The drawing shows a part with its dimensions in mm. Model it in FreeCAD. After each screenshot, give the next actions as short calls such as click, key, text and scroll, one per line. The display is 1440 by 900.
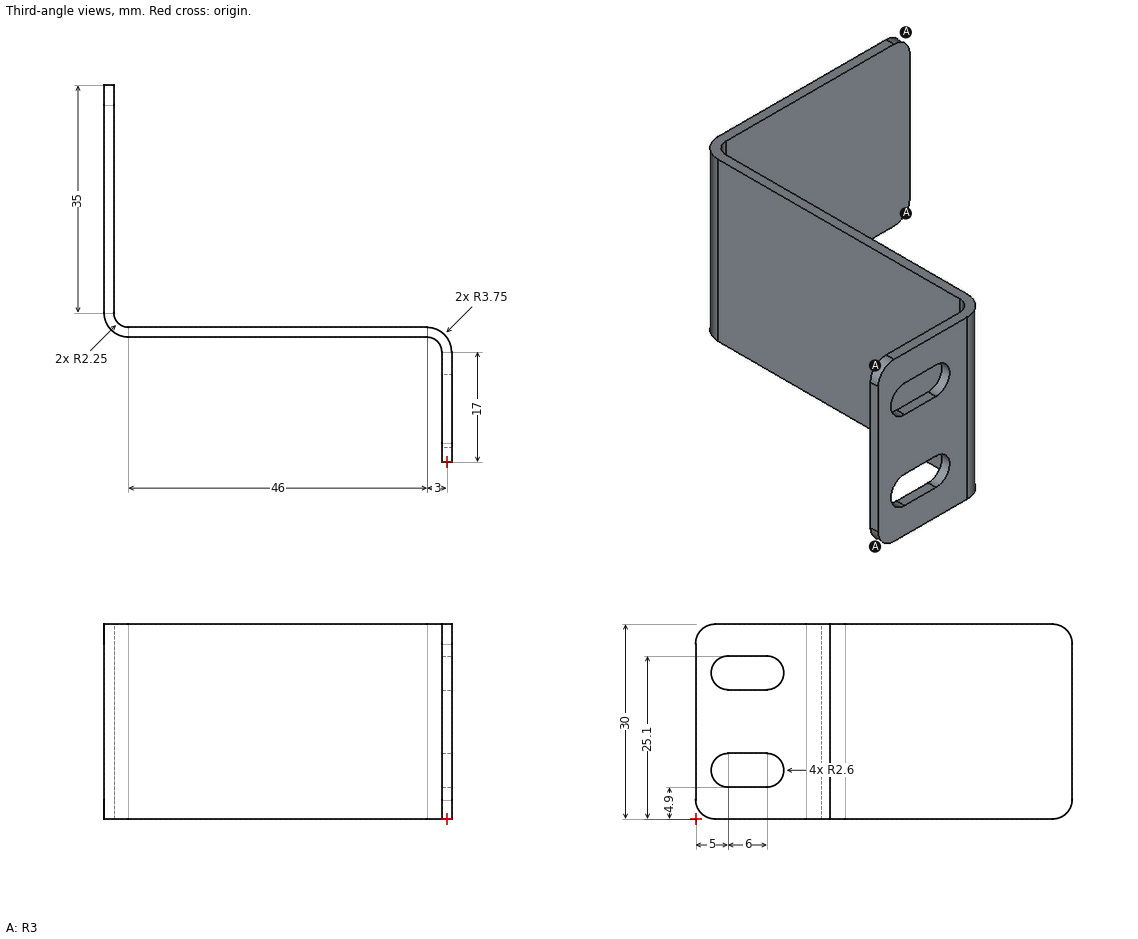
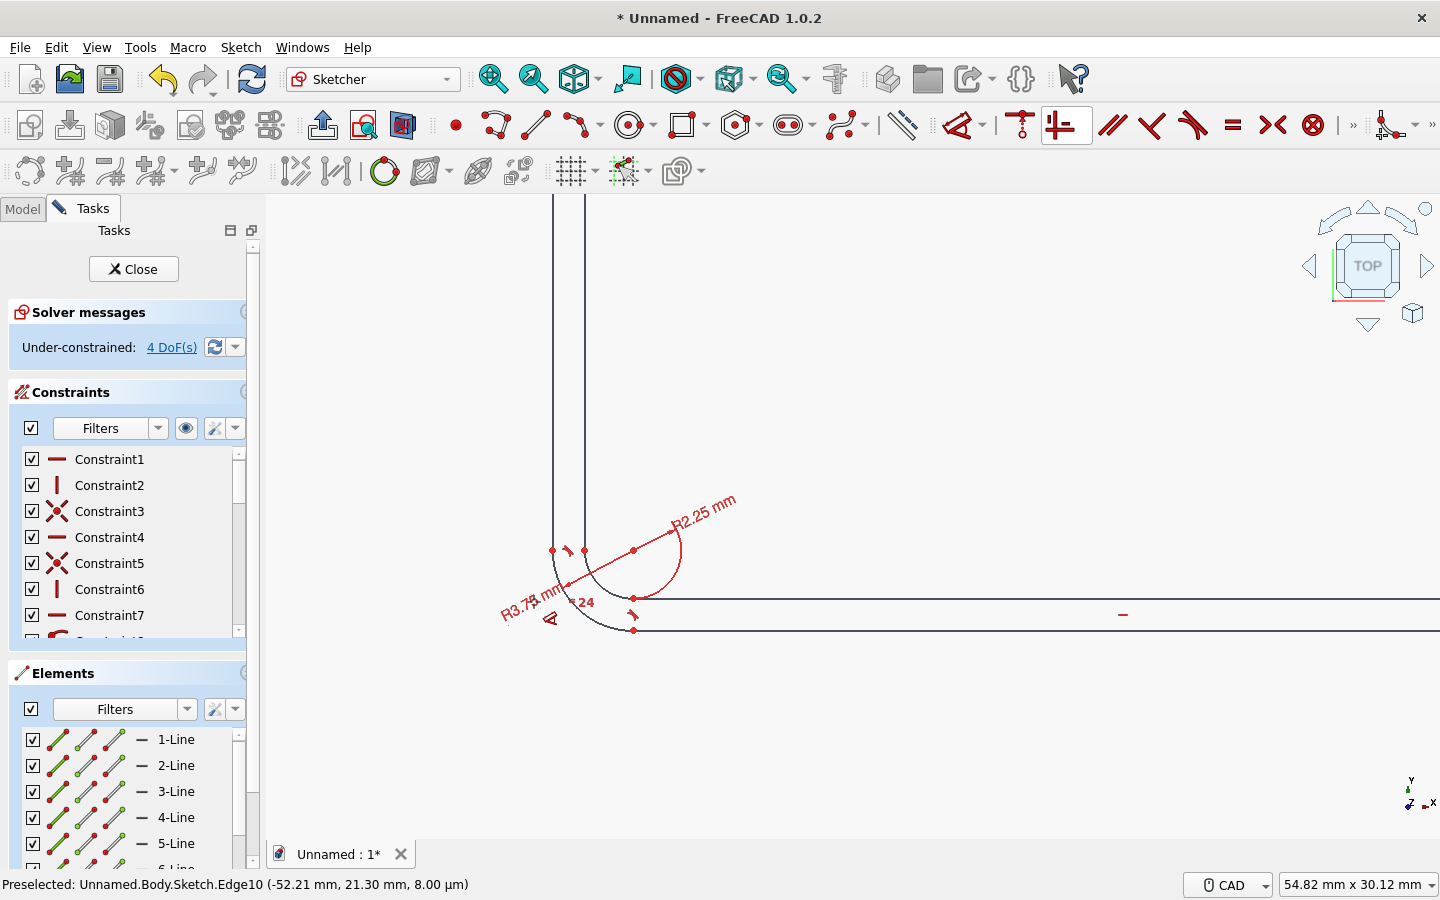
click(927, 599)
click(954, 565)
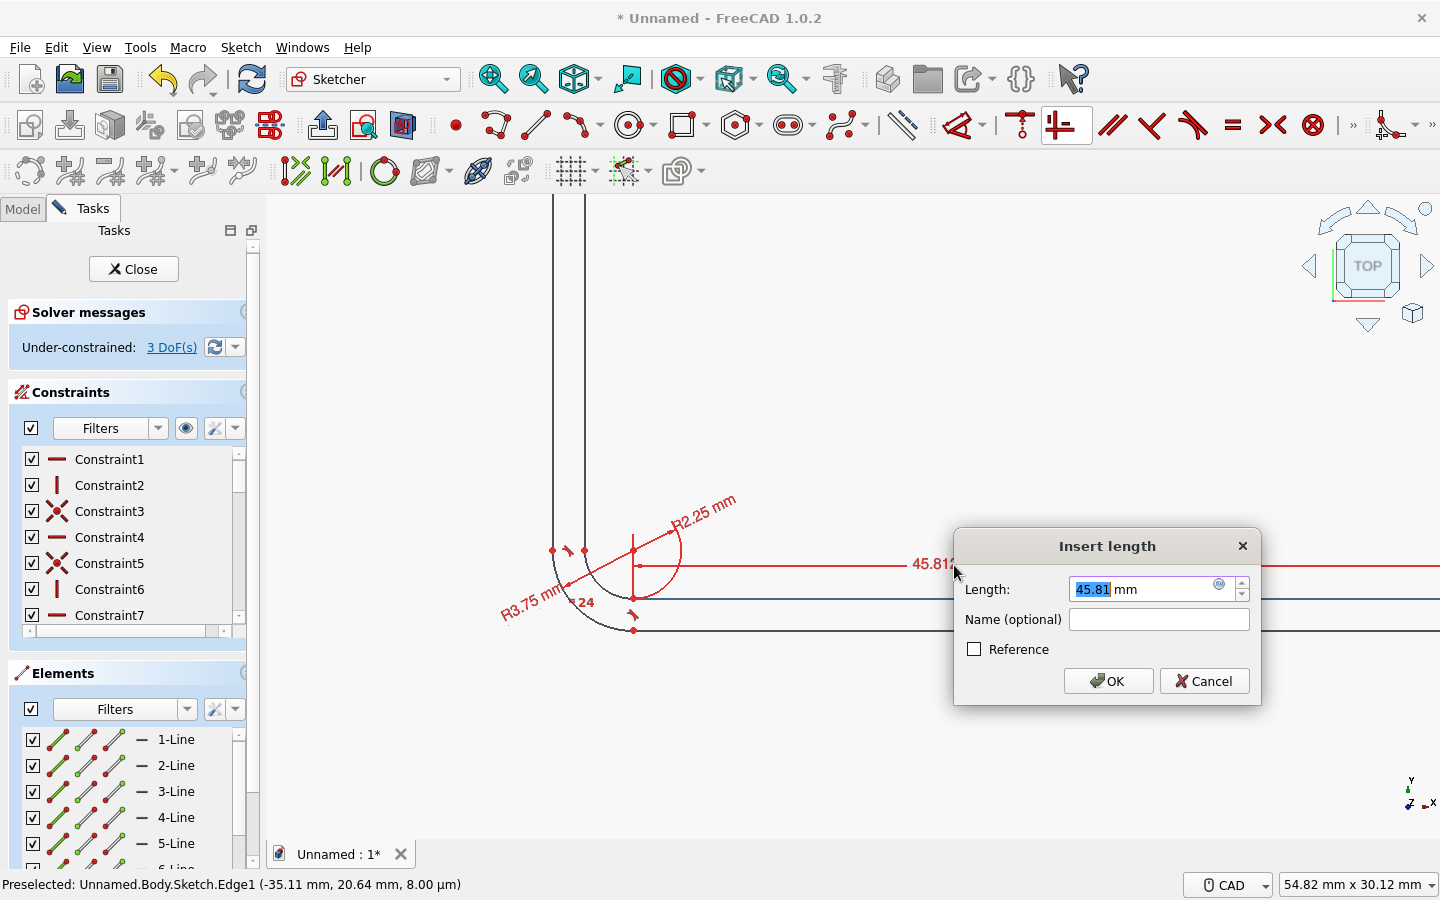
text(46)
key(Return)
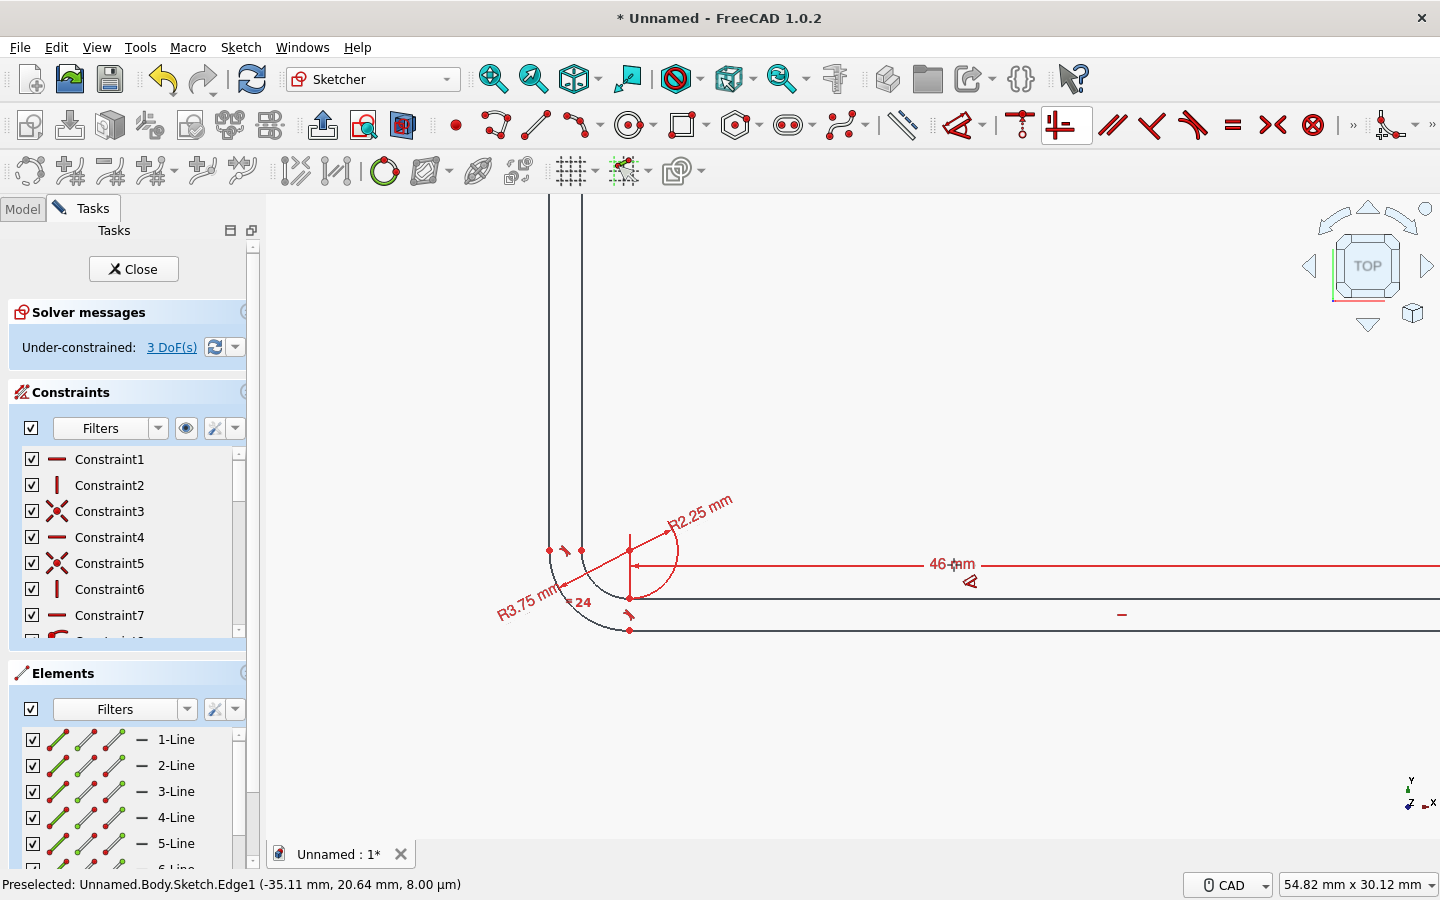
click(582, 326)
click(616, 386)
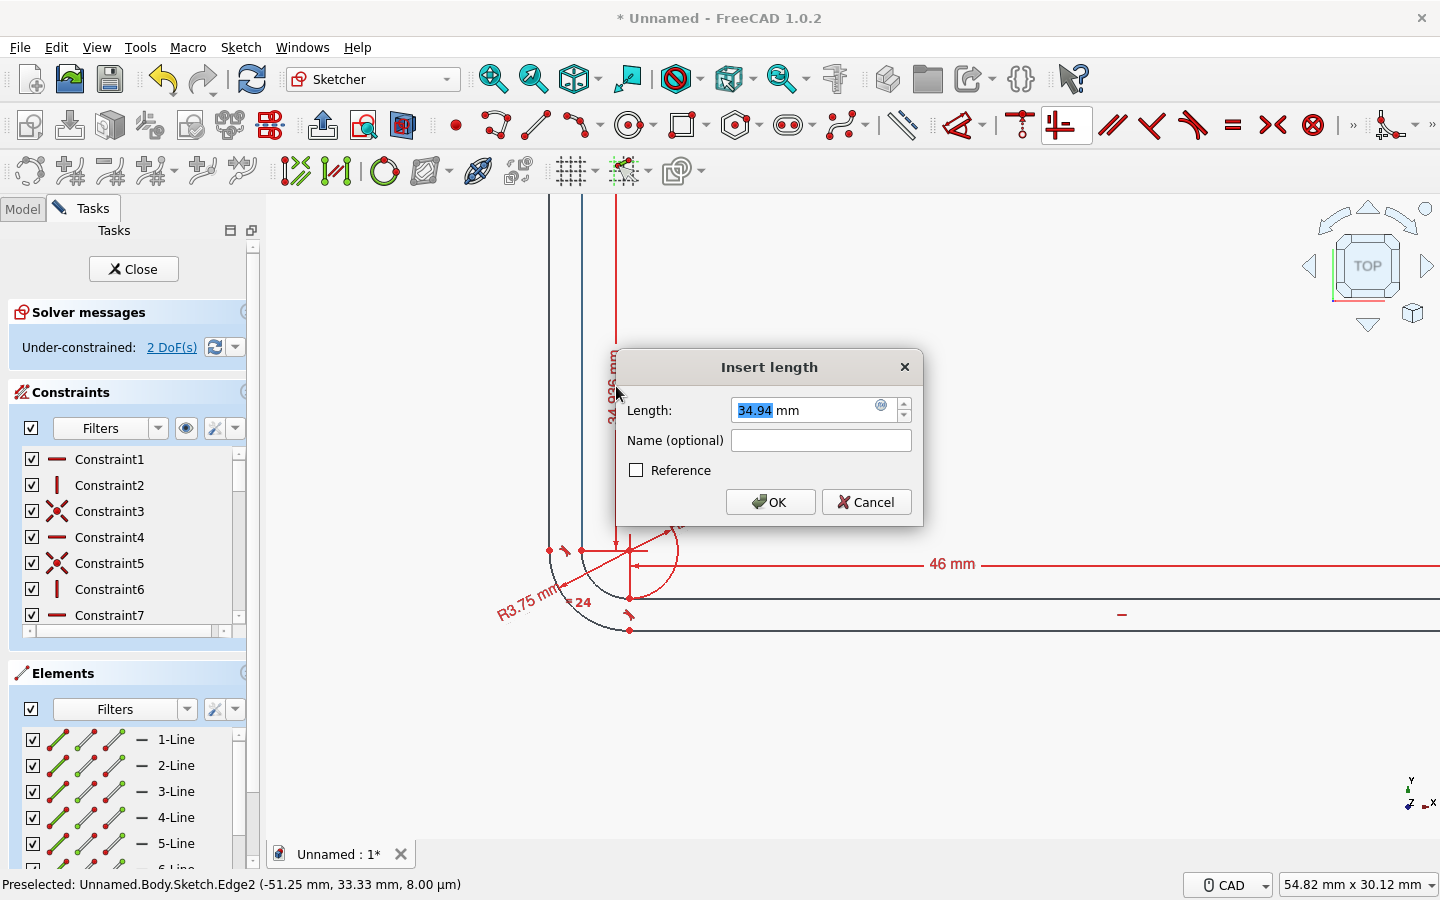
text(35)
key(Return)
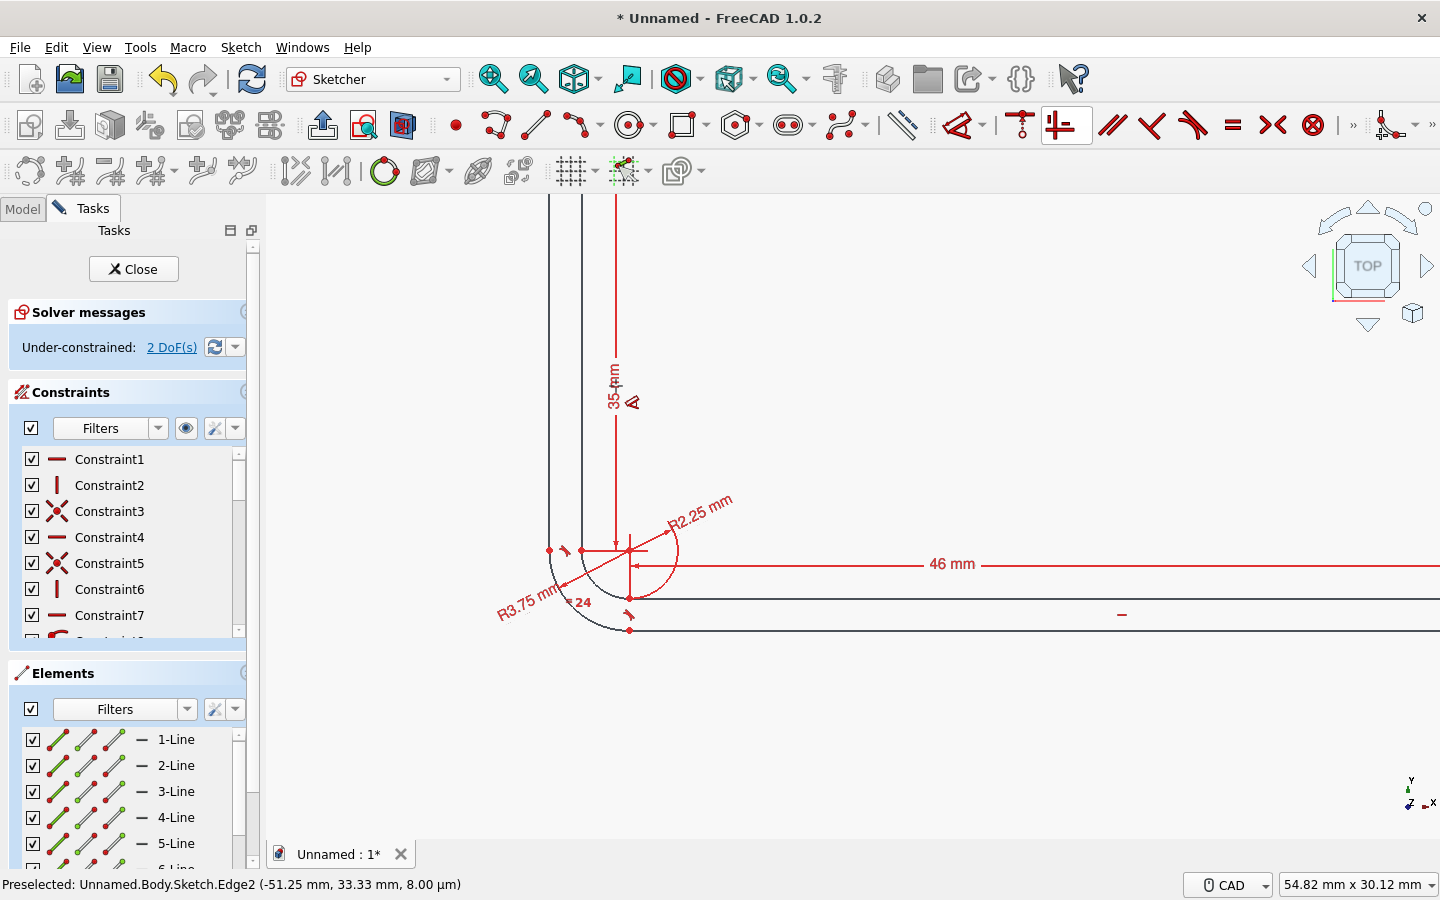
scroll(588, 573, down, 5)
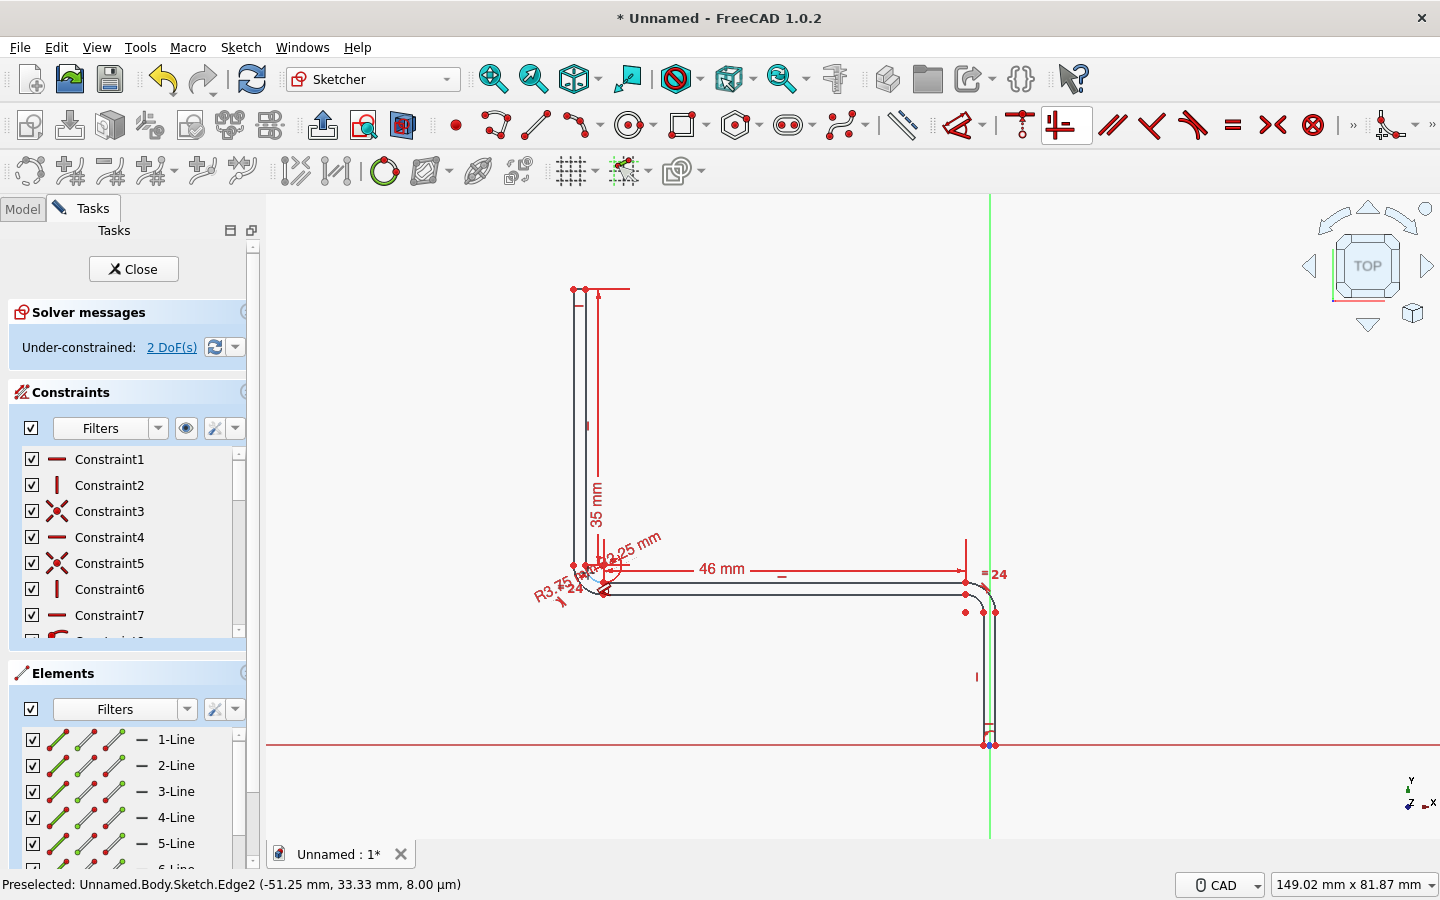
scroll(984, 652, up, 5)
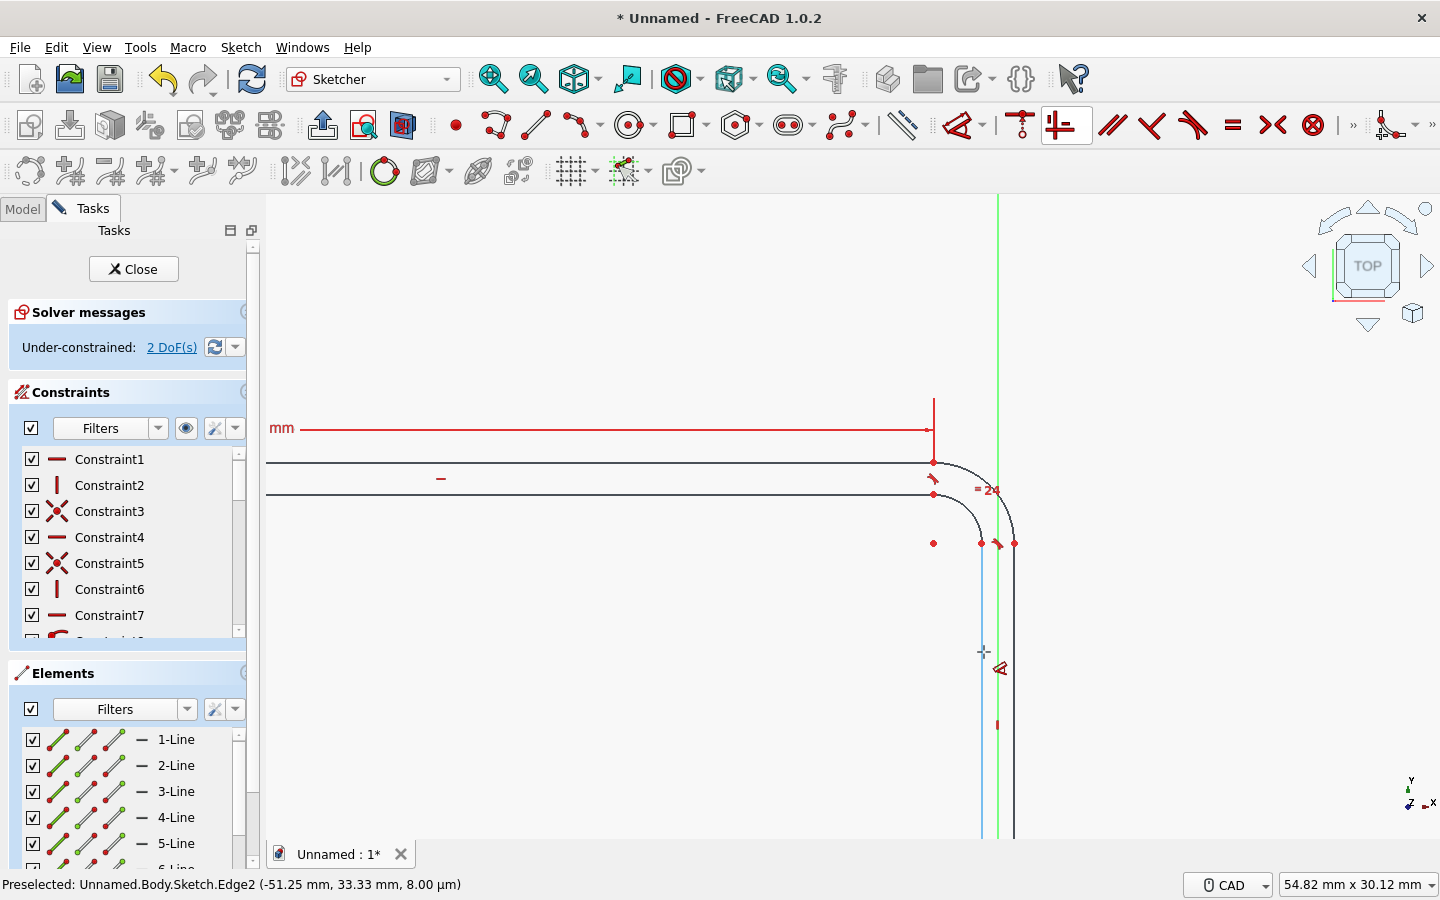
click(982, 652)
click(948, 677)